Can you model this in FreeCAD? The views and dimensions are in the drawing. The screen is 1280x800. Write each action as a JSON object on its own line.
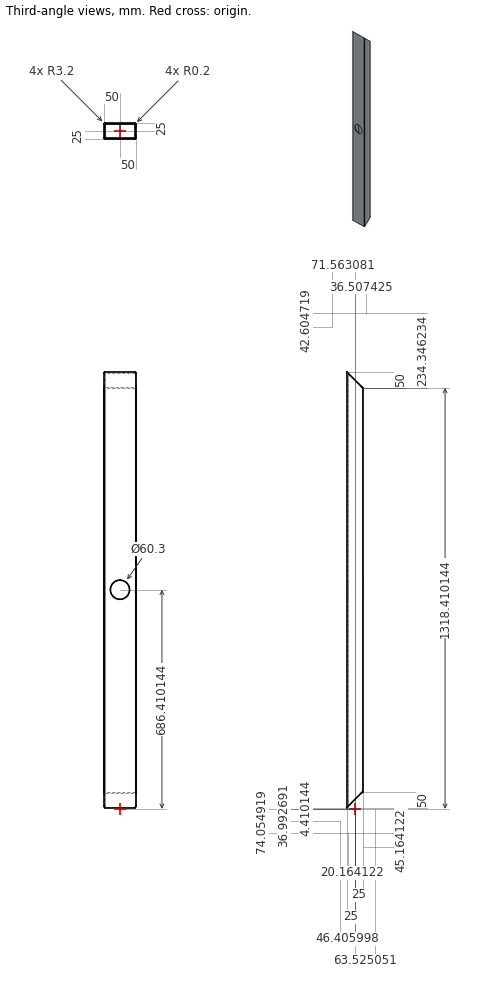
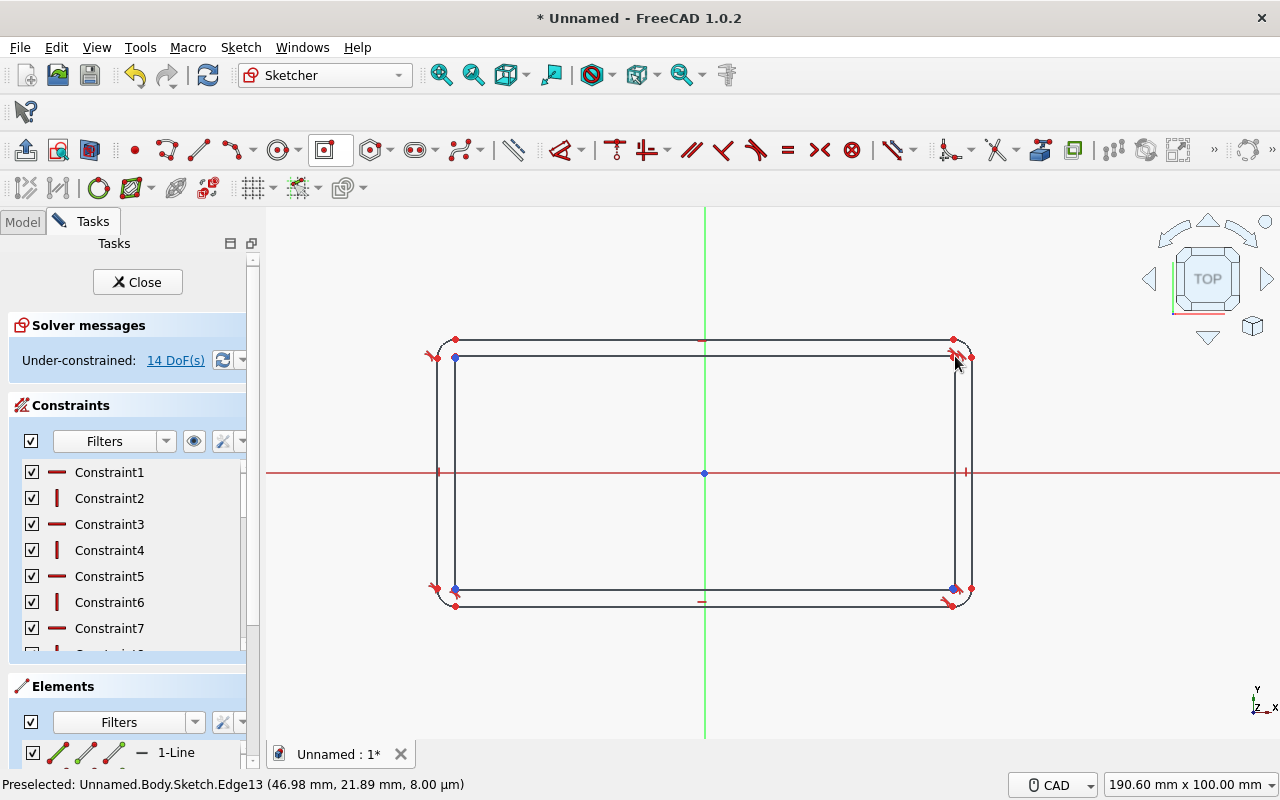
{"action": "scroll", "coordinate": [961, 605], "scroll_direction": "up", "scroll_amount": 3}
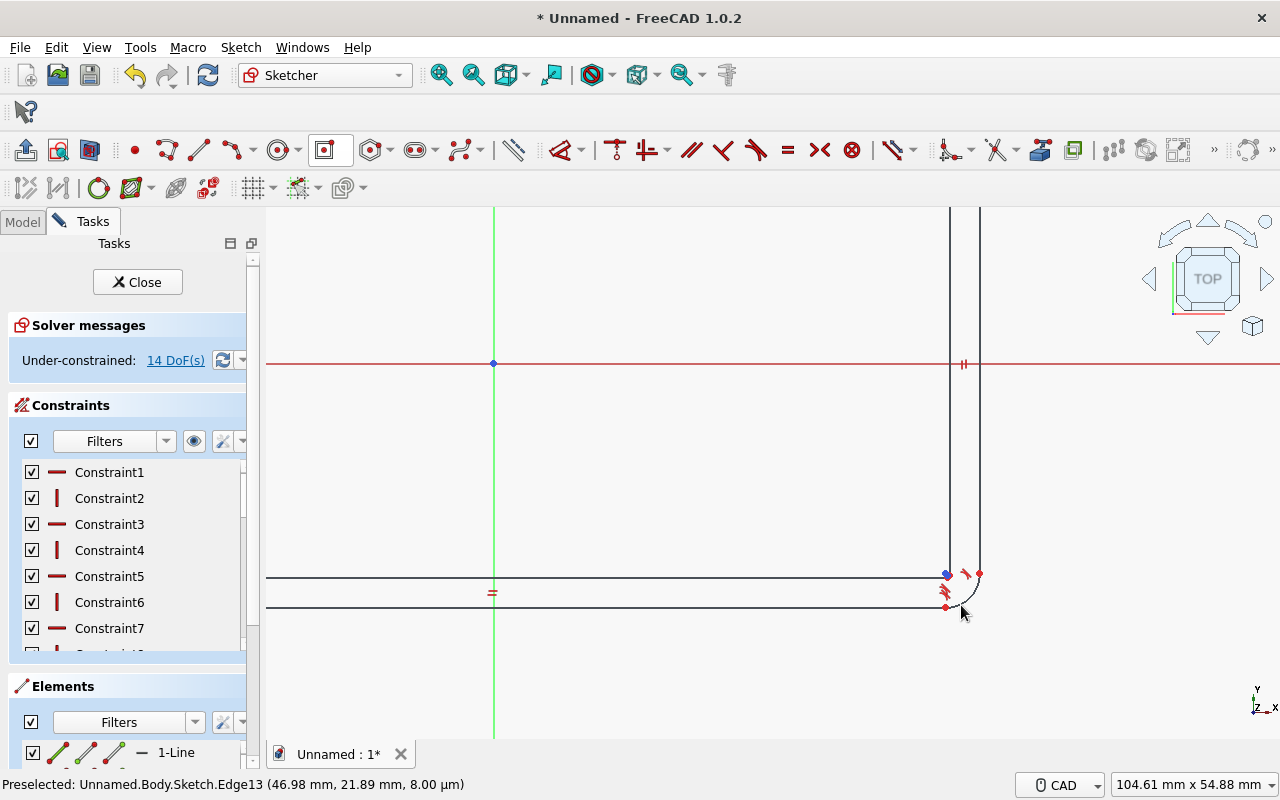
{"action": "left_click", "coordinate": [961, 604]}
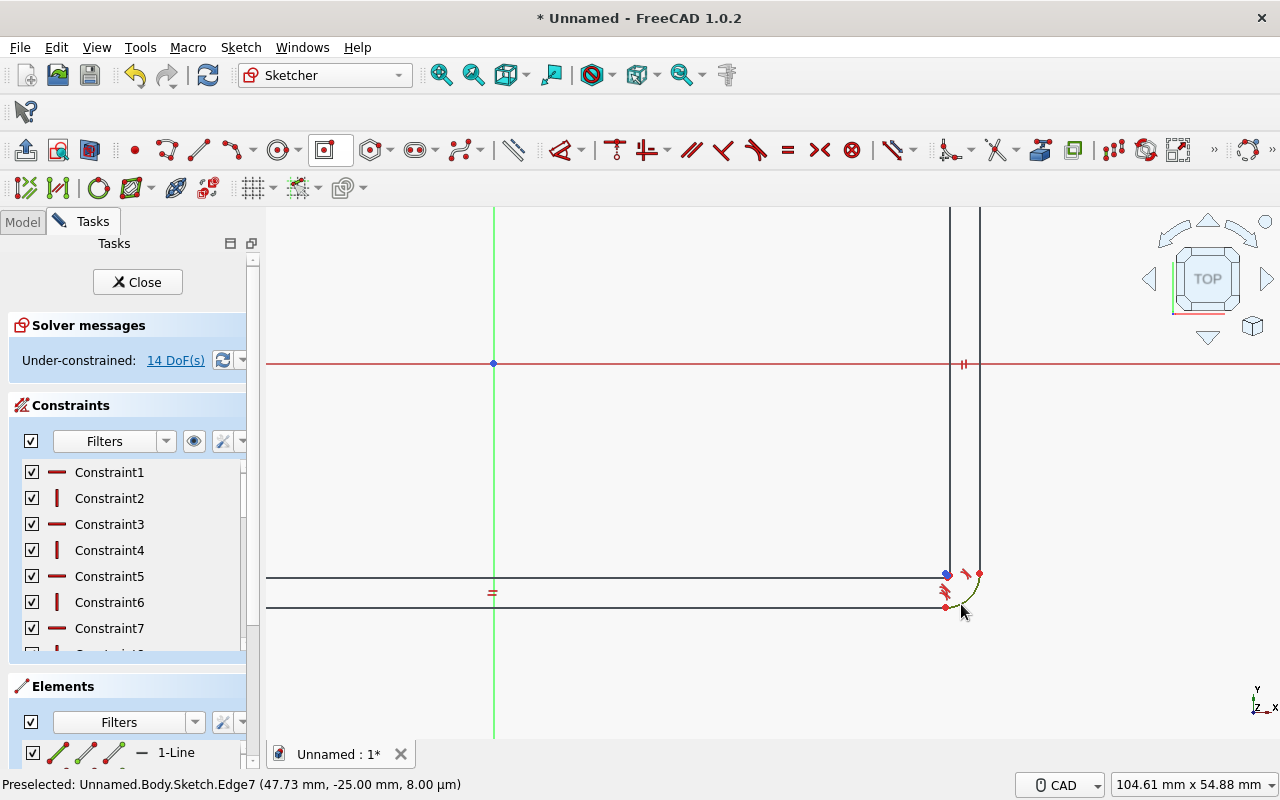
{"action": "scroll", "coordinate": [949, 577], "scroll_direction": "up", "scroll_amount": 11}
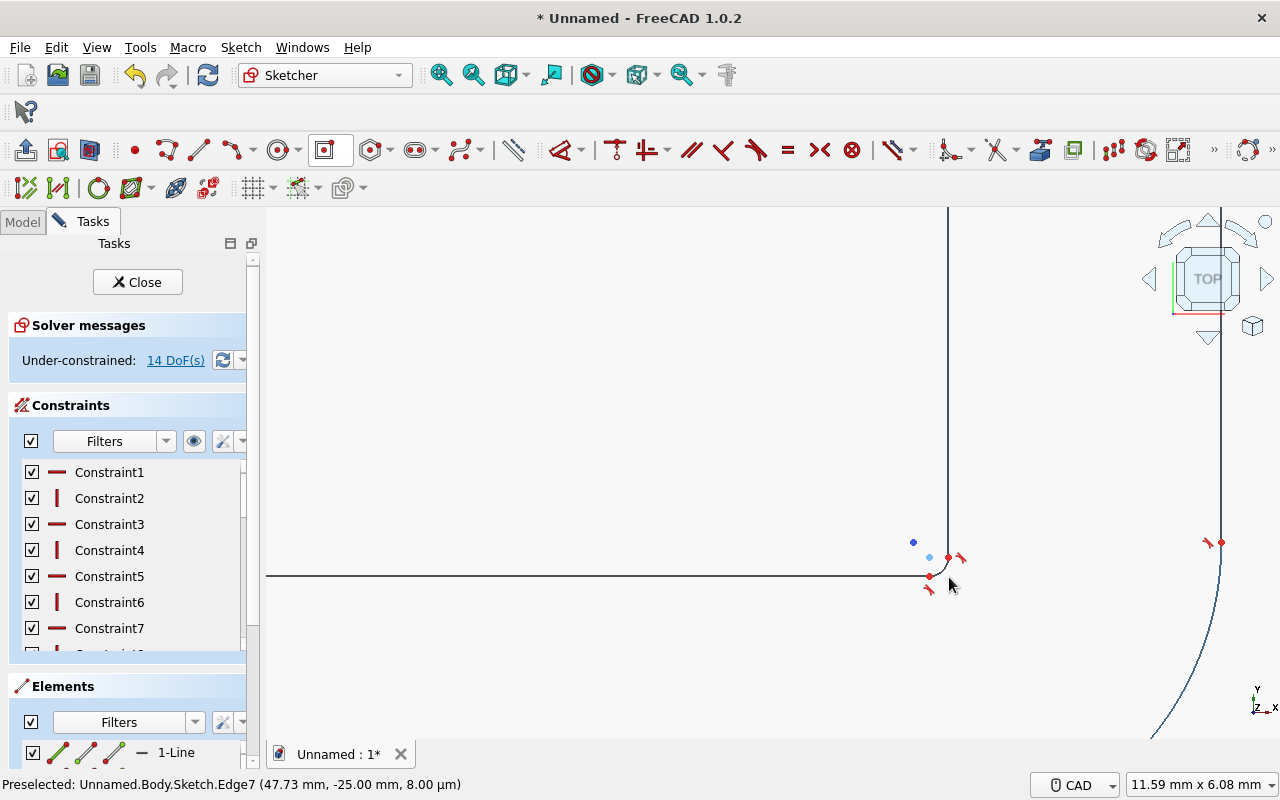
{"action": "left_click", "coordinate": [943, 571]}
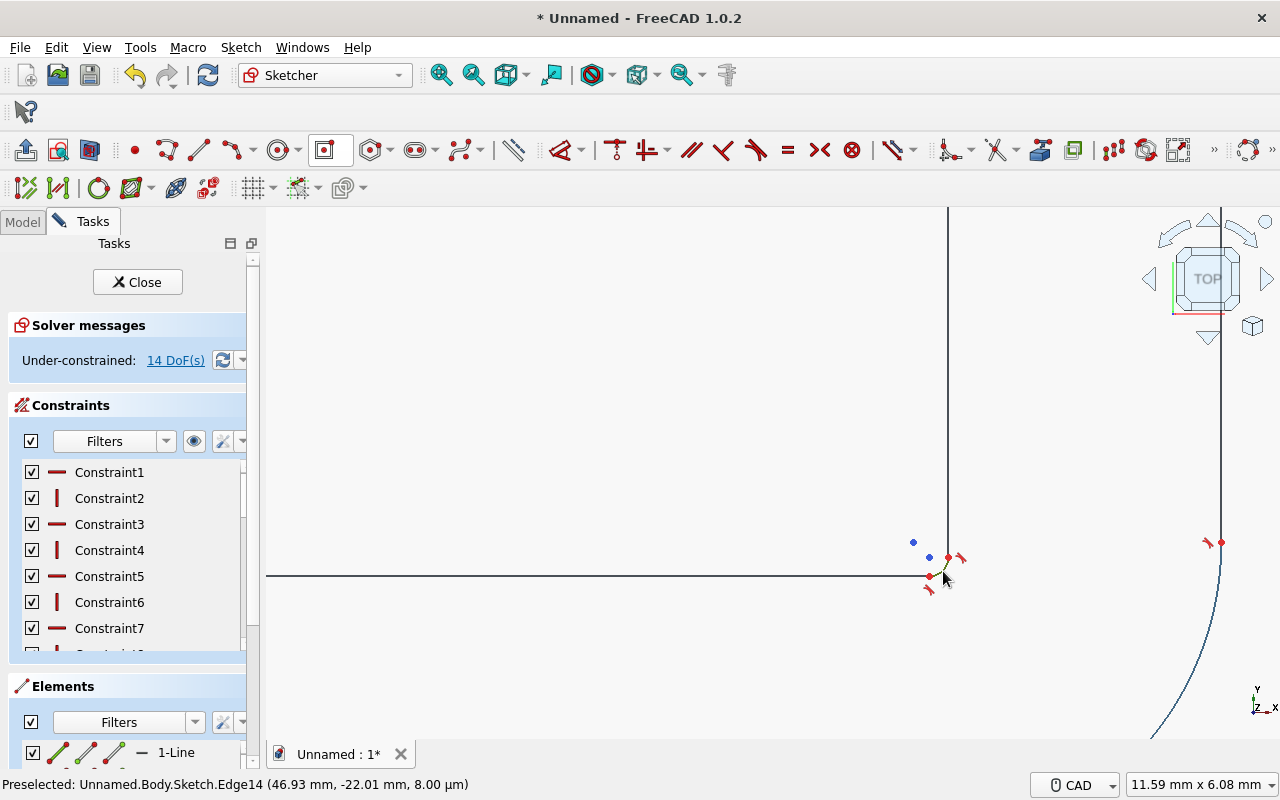
{"action": "key", "text": "c"}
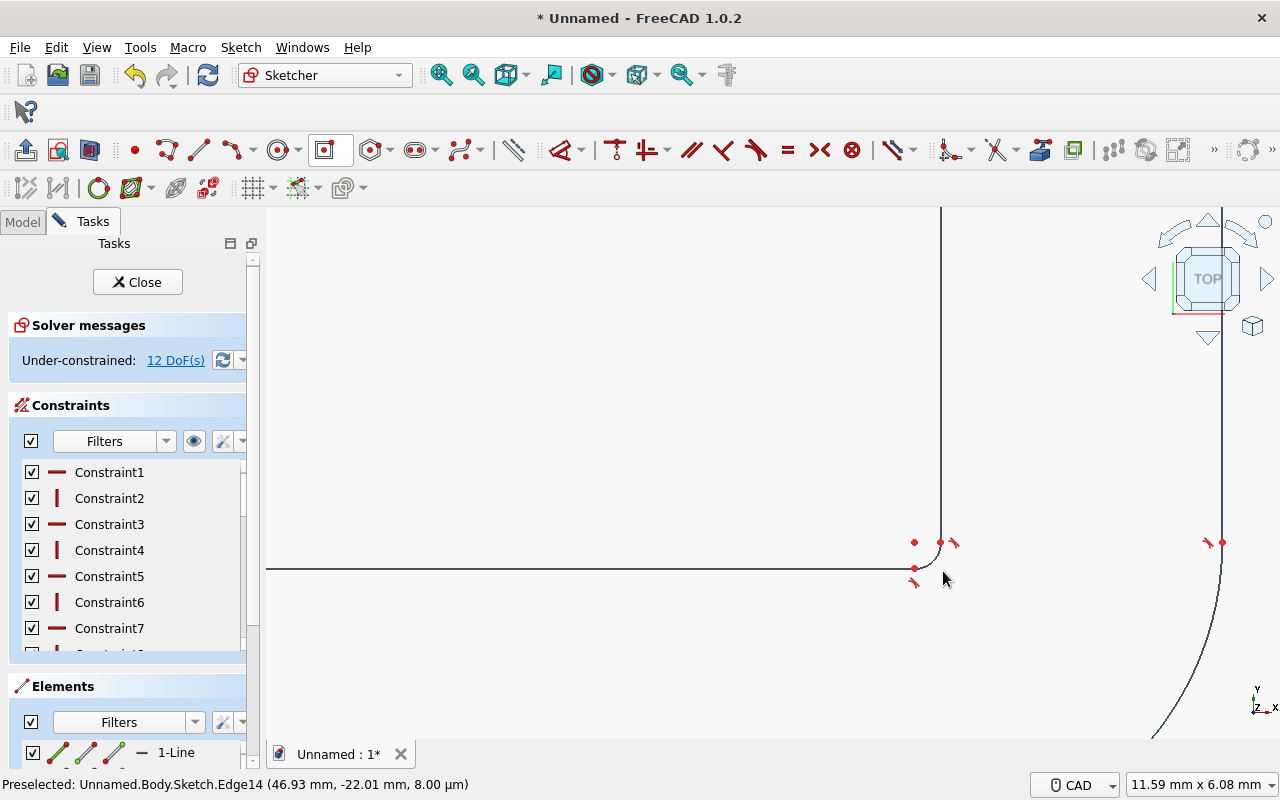
{"action": "scroll", "coordinate": [955, 591], "scroll_direction": "down", "scroll_amount": 14}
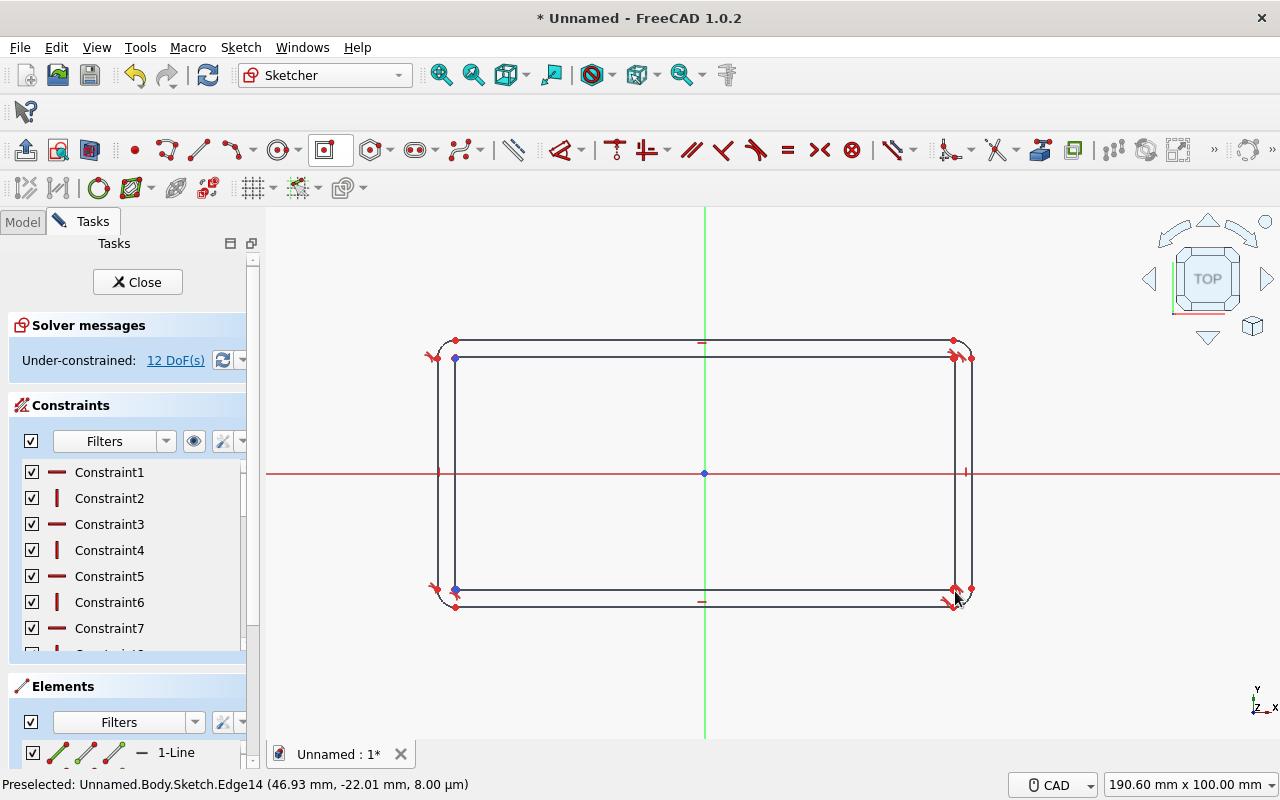
{"action": "scroll", "coordinate": [440, 597], "scroll_direction": "up", "scroll_amount": 3}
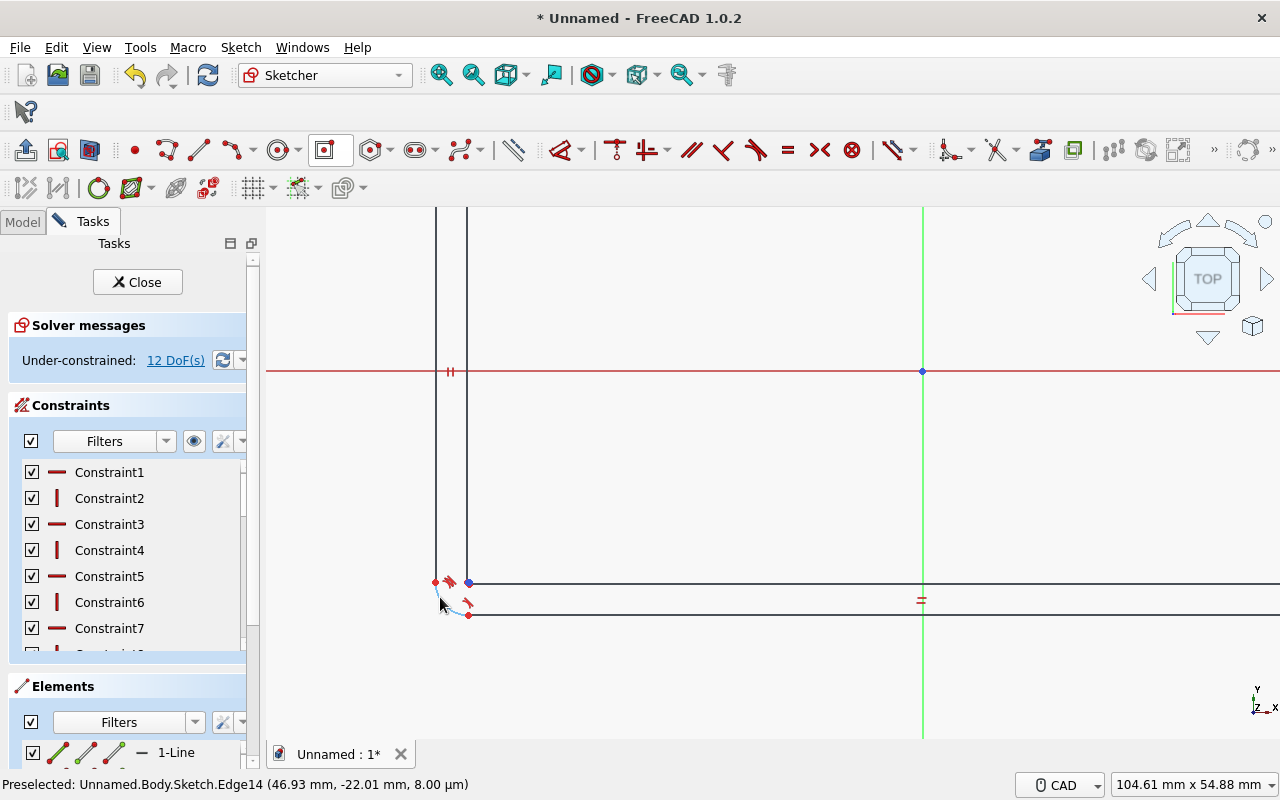
{"action": "left_click", "coordinate": [439, 597]}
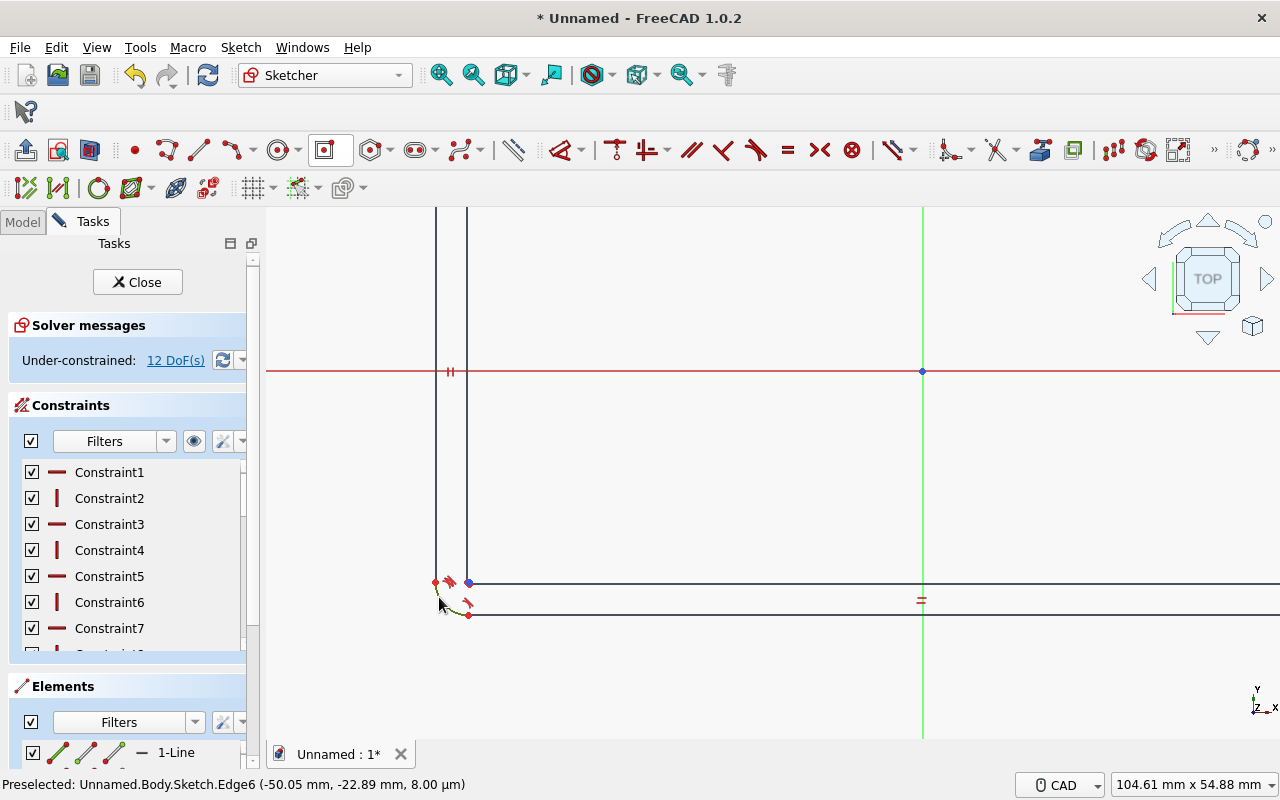
{"action": "scroll", "coordinate": [468, 584], "scroll_direction": "up", "scroll_amount": 11}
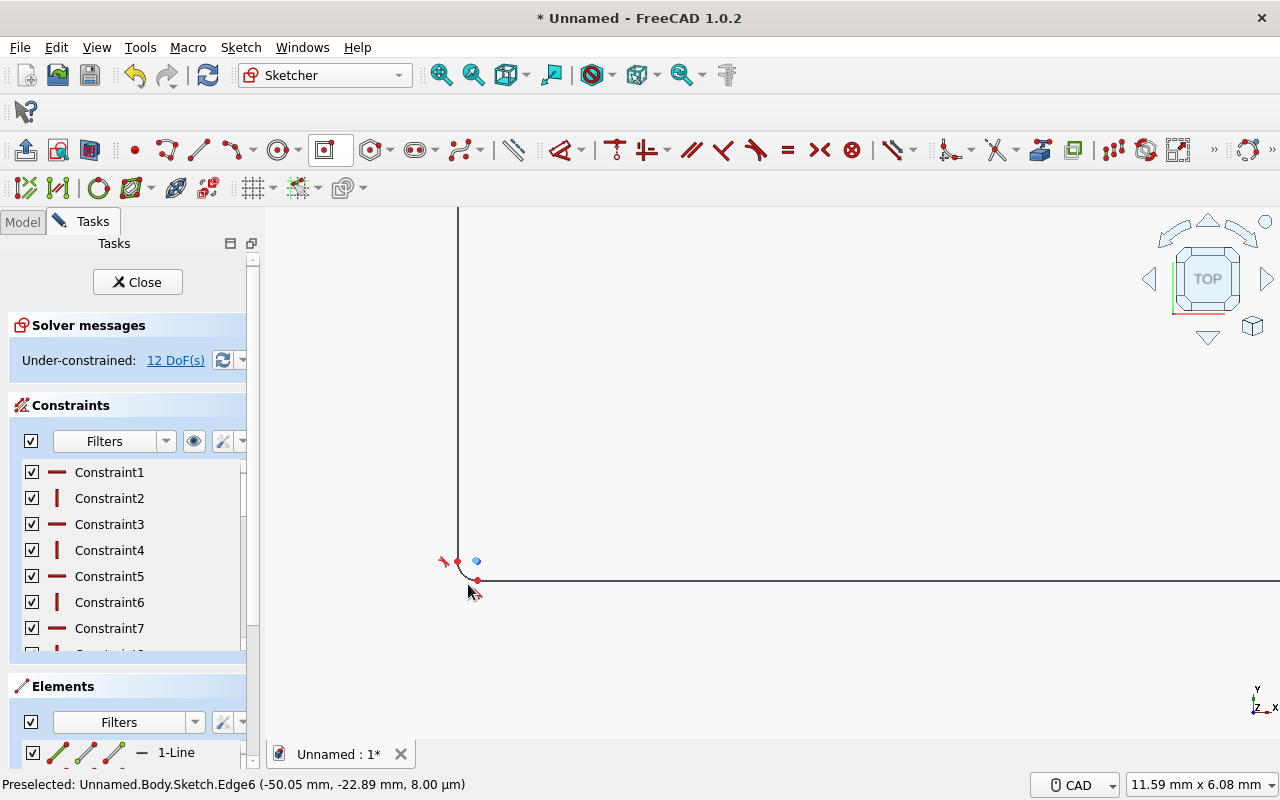
{"action": "left_click", "coordinate": [463, 575]}